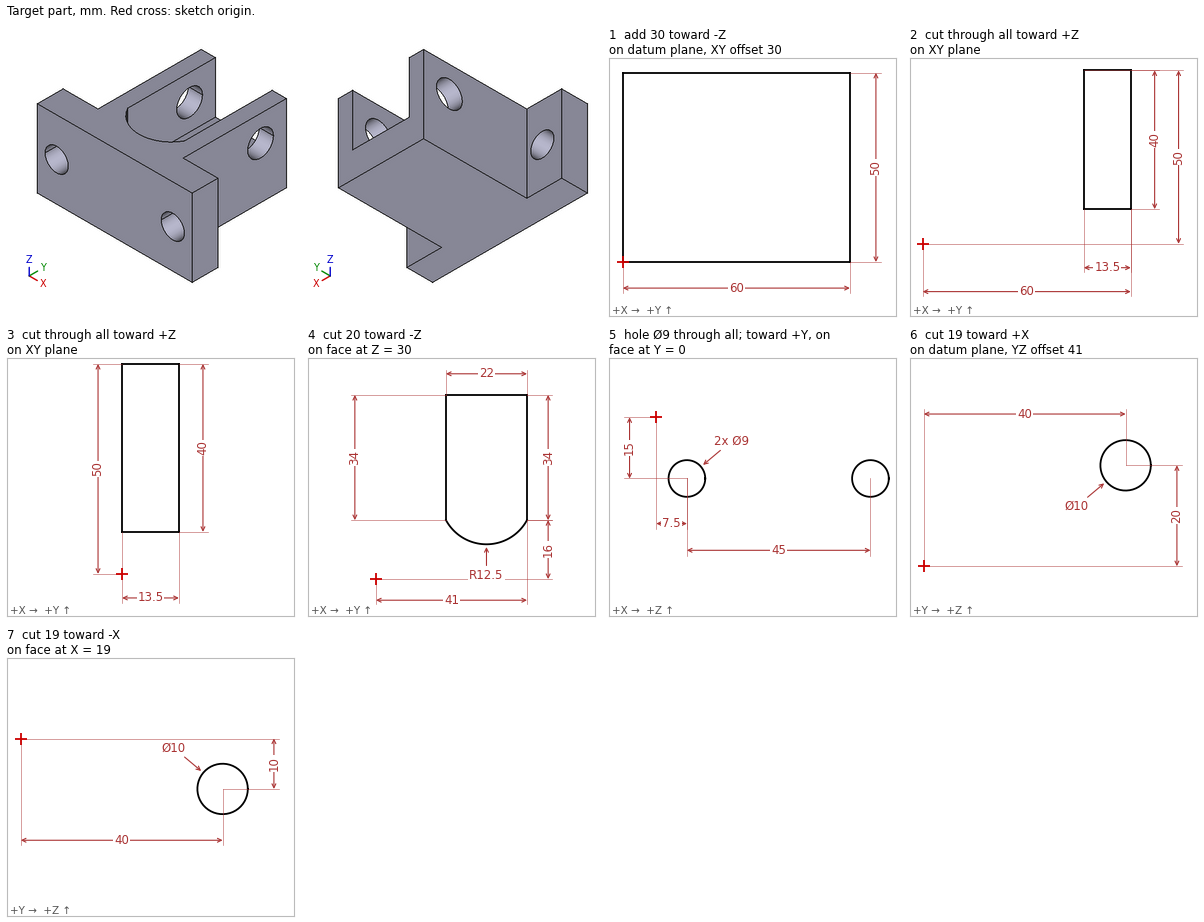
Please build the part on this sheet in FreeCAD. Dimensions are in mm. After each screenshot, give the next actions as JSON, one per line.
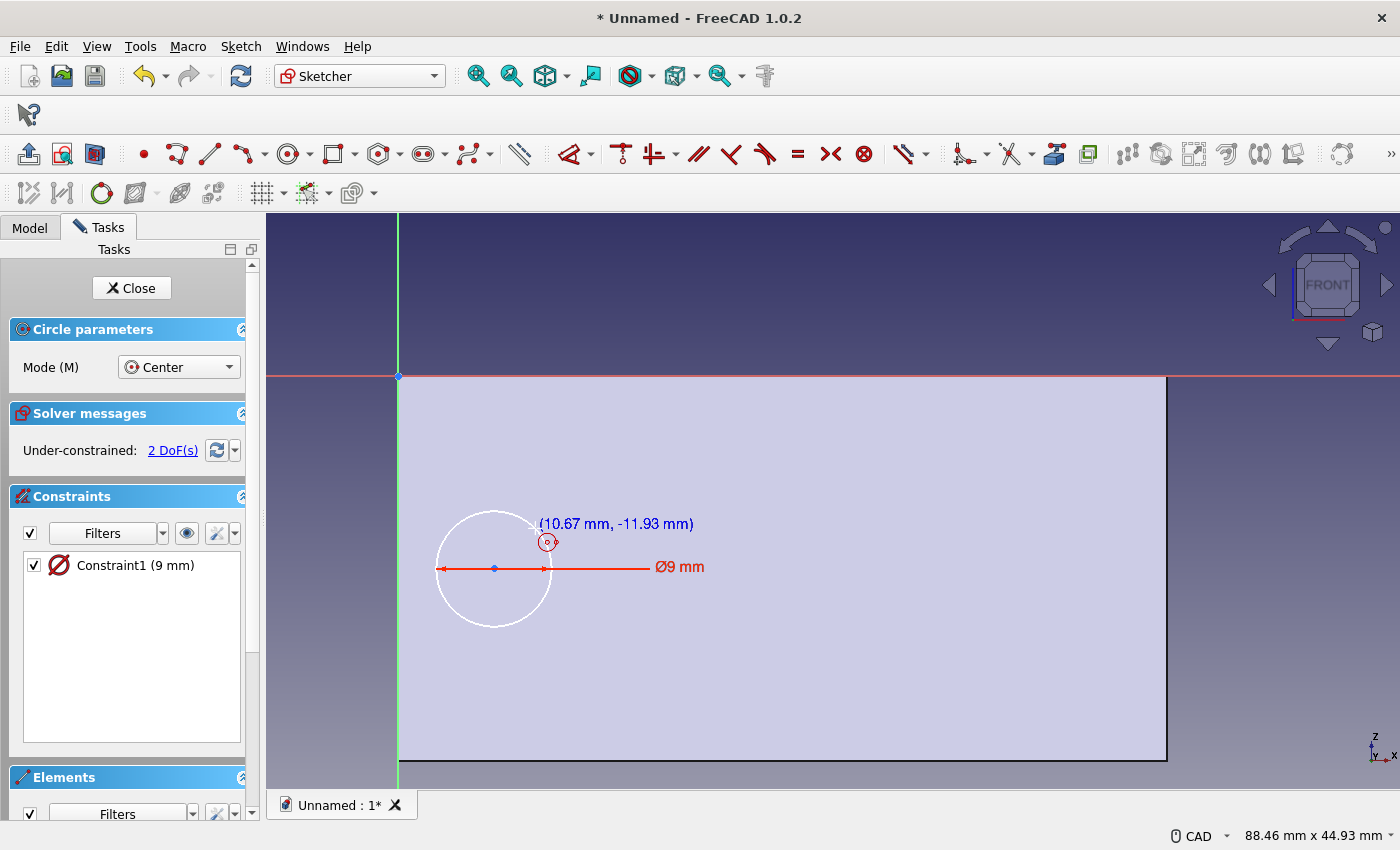
{"action": "left_click", "coordinate": [1071, 568]}
{"action": "mouse_move", "coordinate": [1112, 528]}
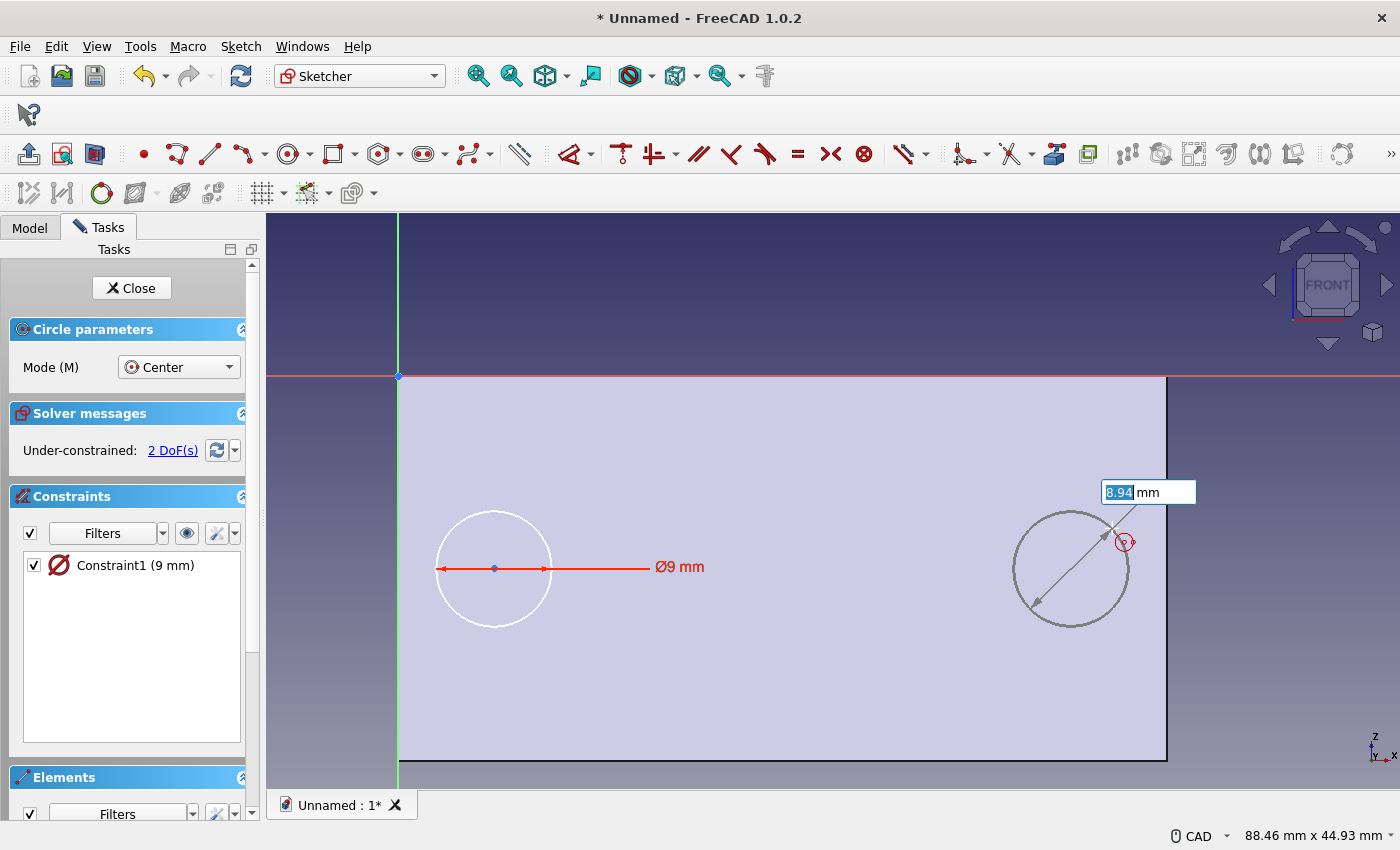
{"action": "type", "text": "9"}
{"action": "key", "text": "Return"}
{"action": "key", "text": "Escape"}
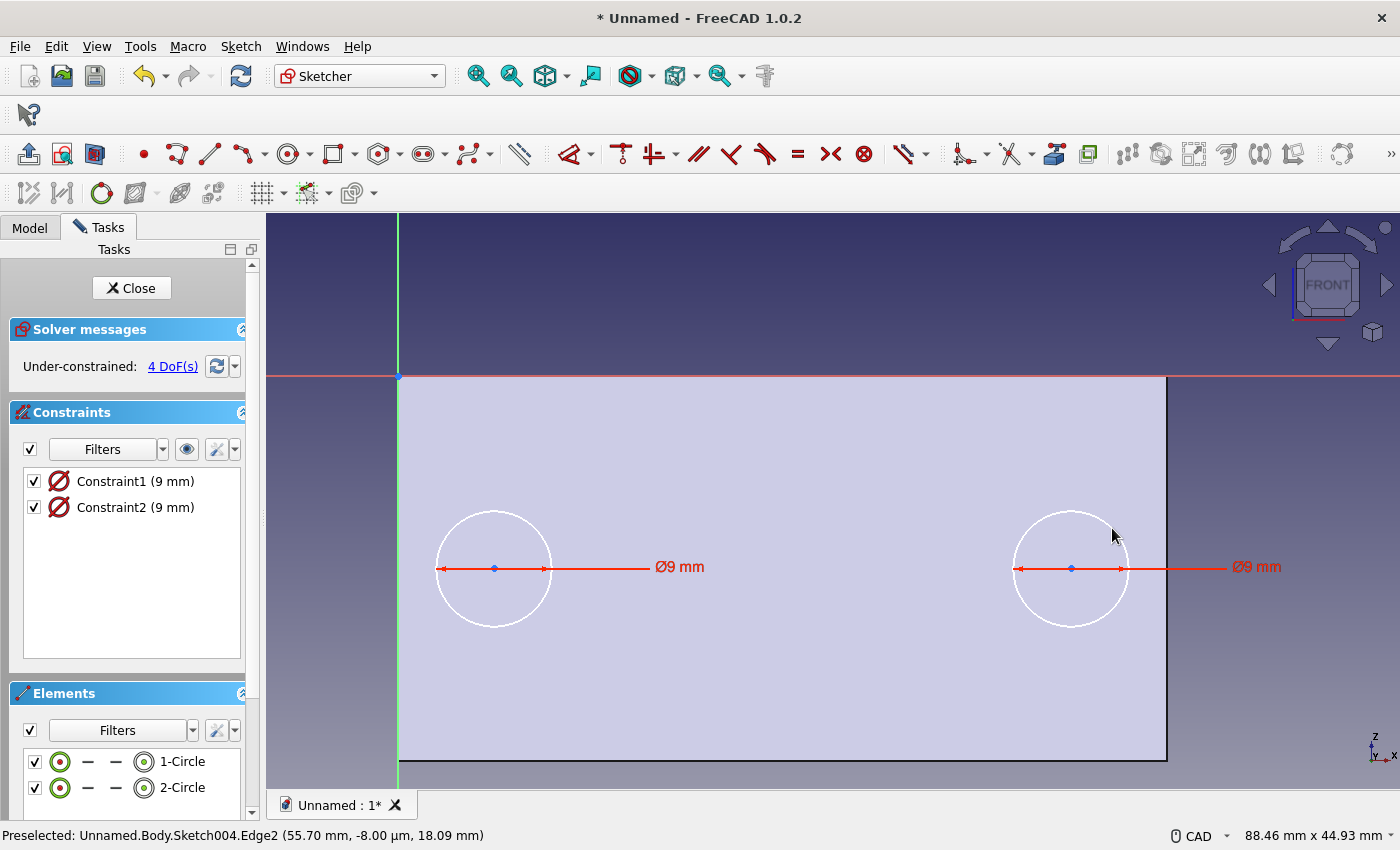
{"action": "left_click", "coordinate": [494, 569]}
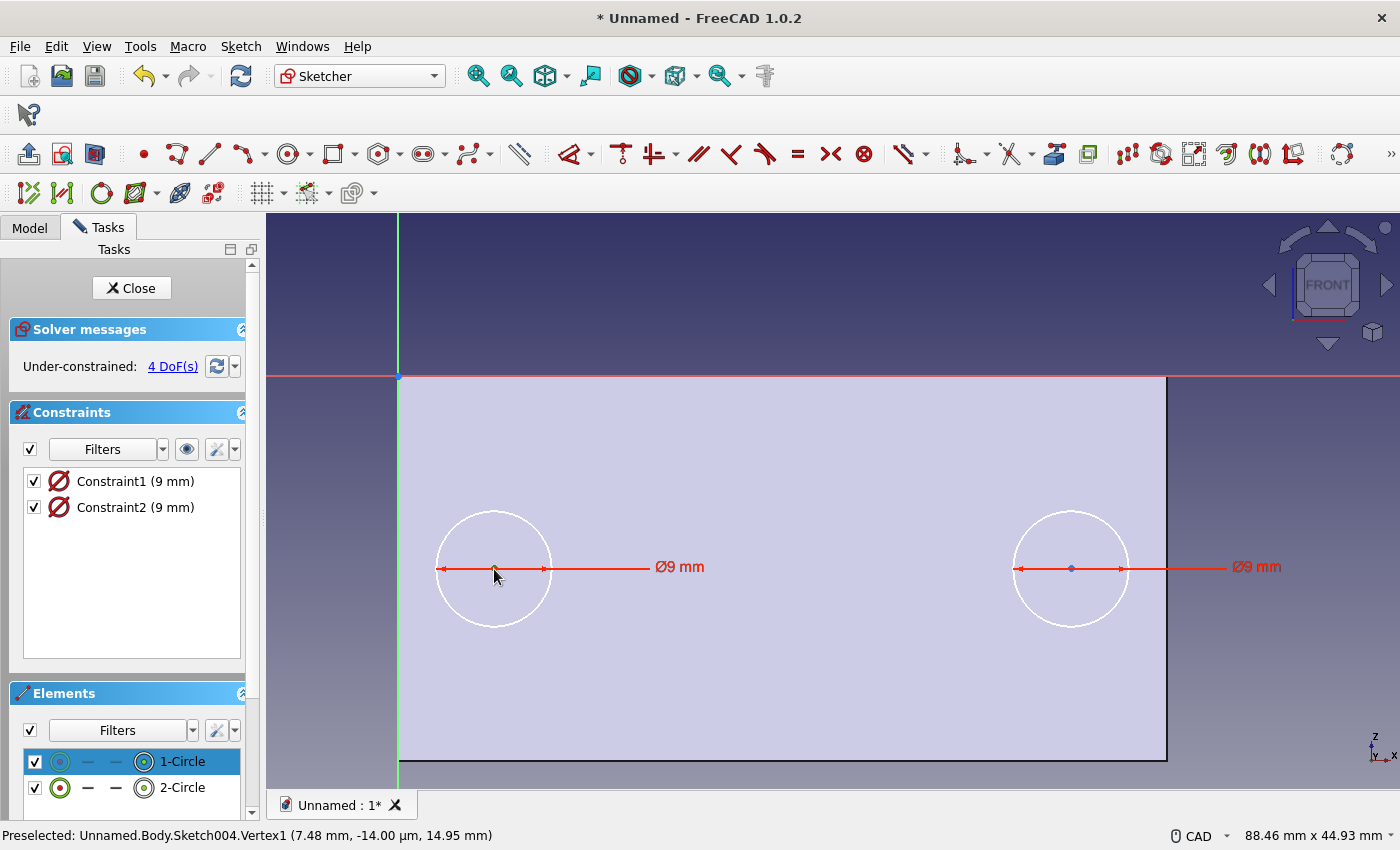
{"action": "left_click", "coordinate": [1071, 569]}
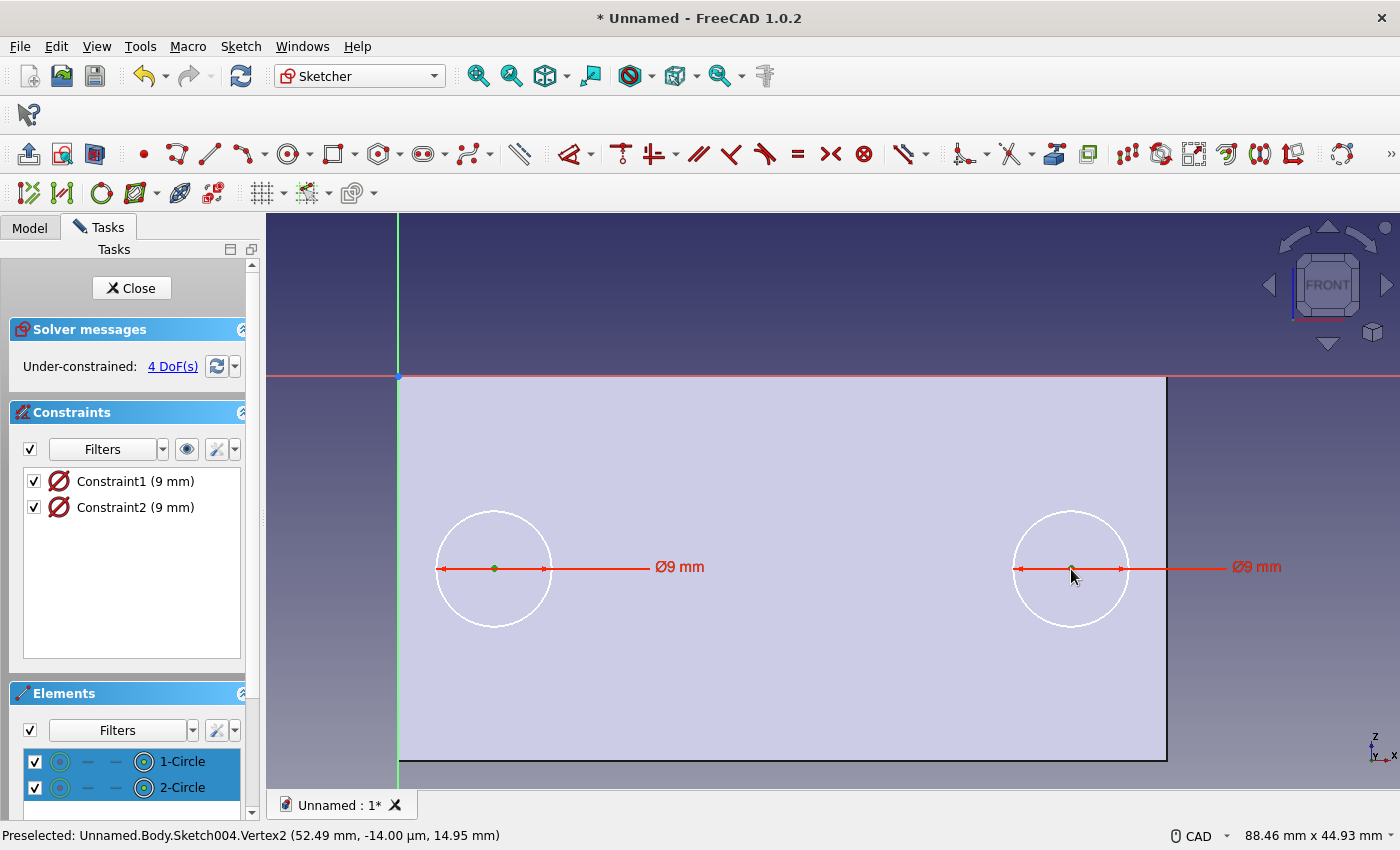
{"action": "left_click", "coordinate": [676, 154]}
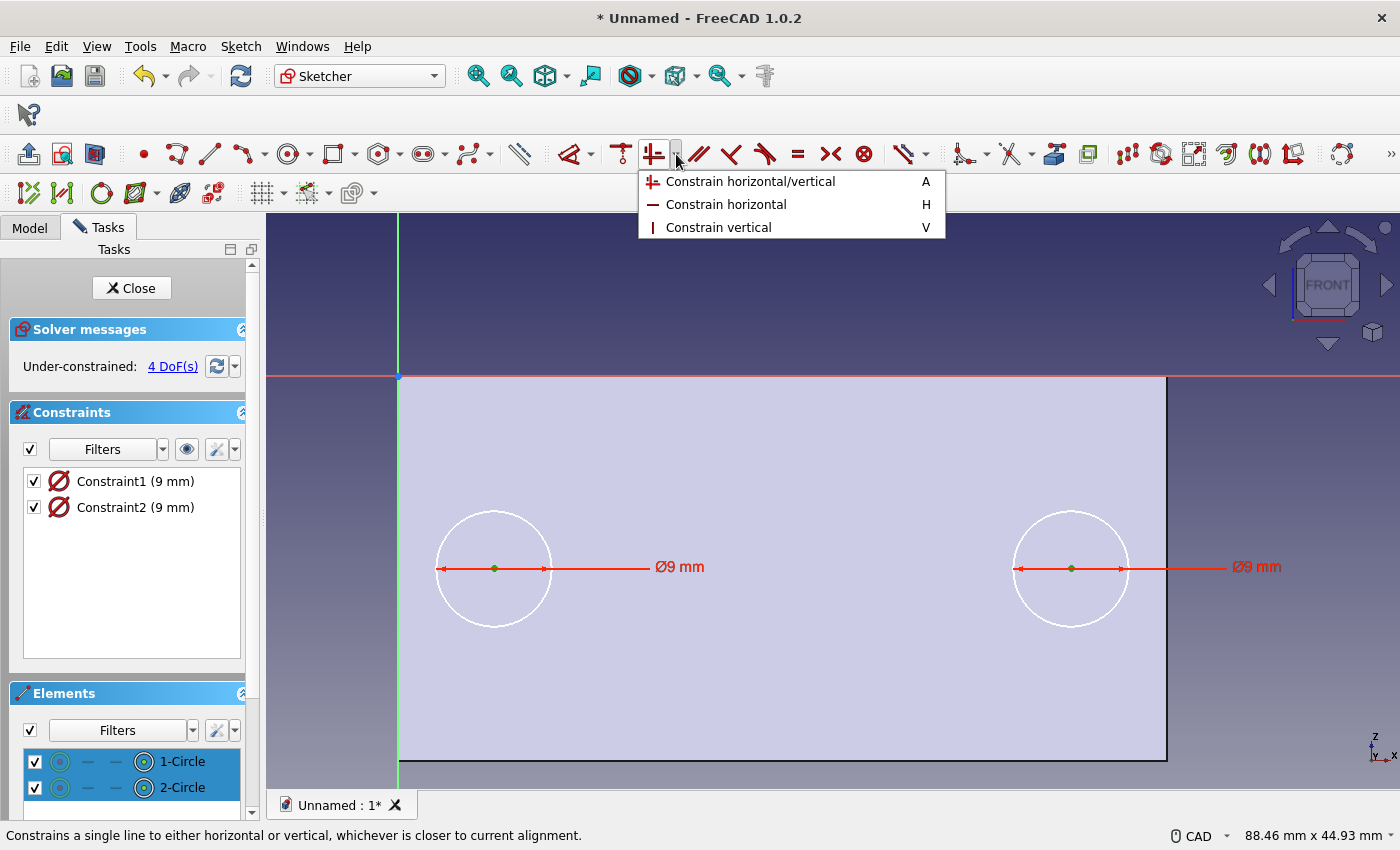
{"action": "left_click", "coordinate": [792, 204]}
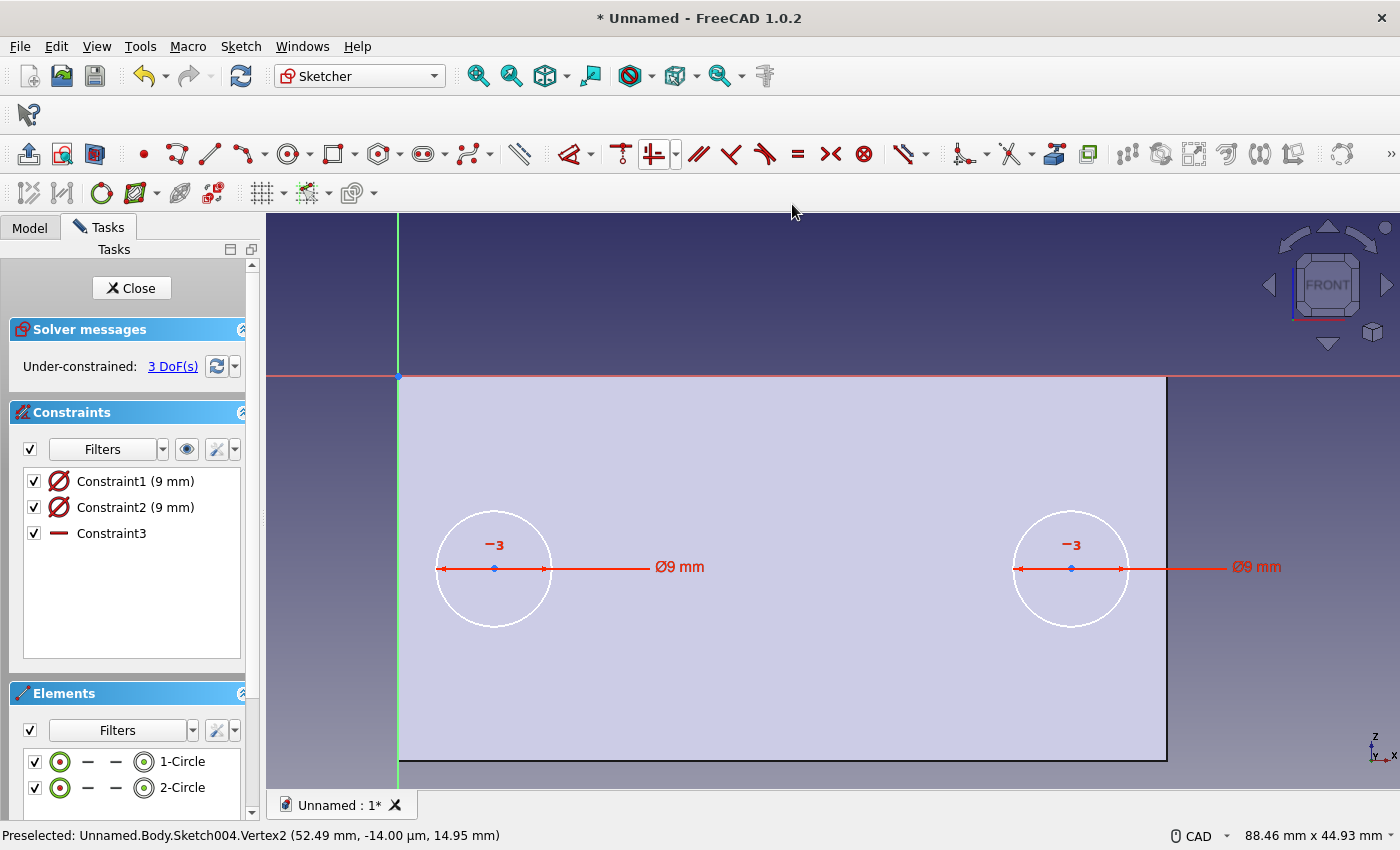
{"action": "left_click", "coordinate": [494, 569]}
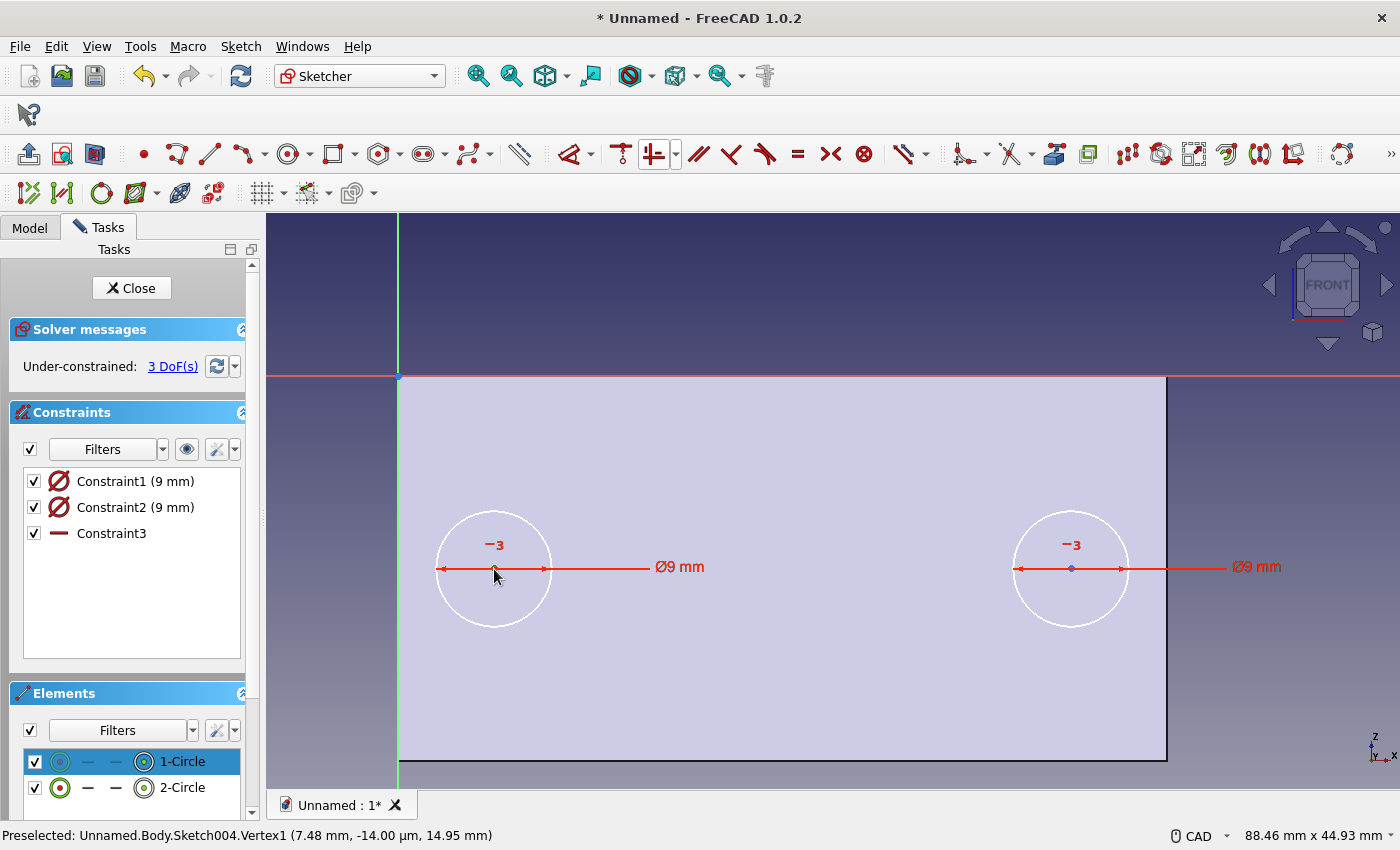
{"action": "key", "text": "i"}